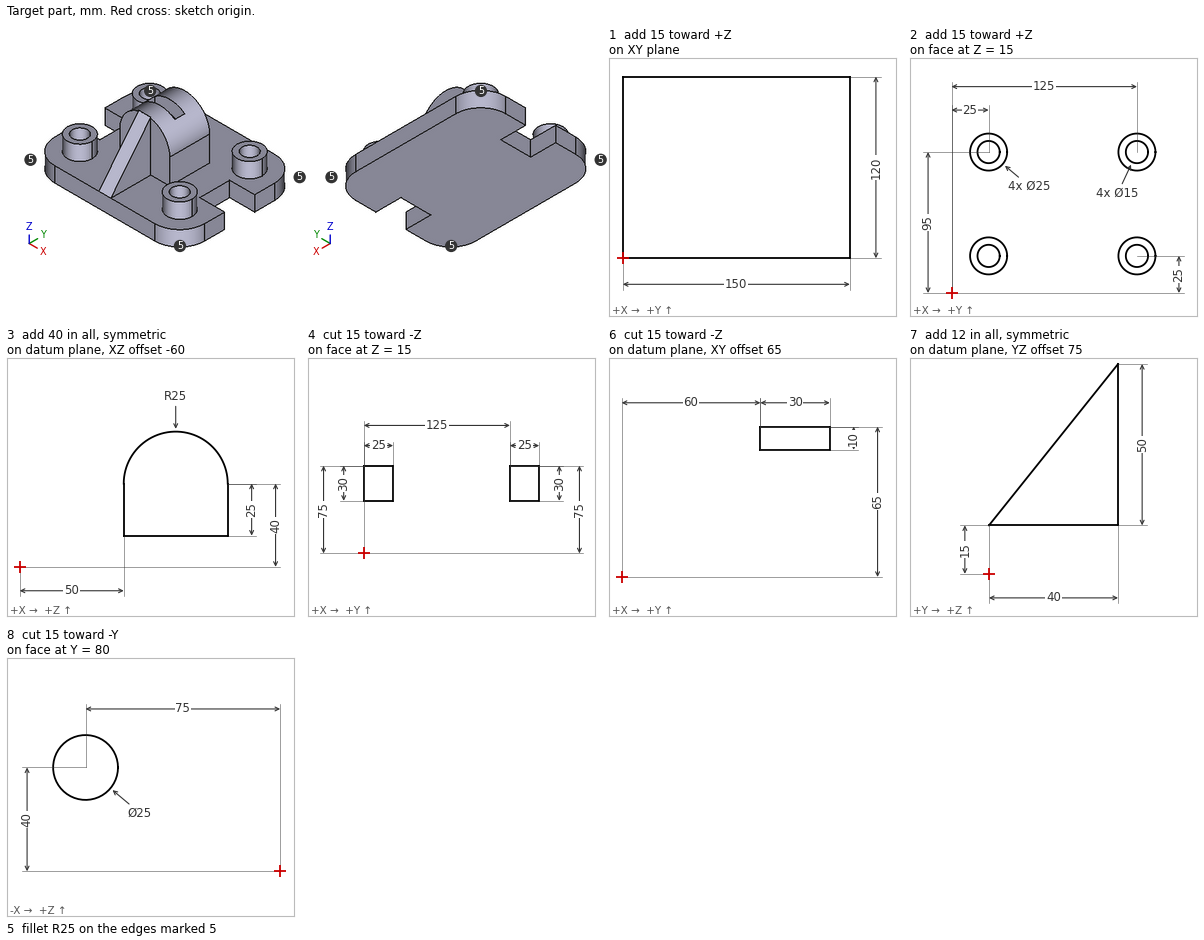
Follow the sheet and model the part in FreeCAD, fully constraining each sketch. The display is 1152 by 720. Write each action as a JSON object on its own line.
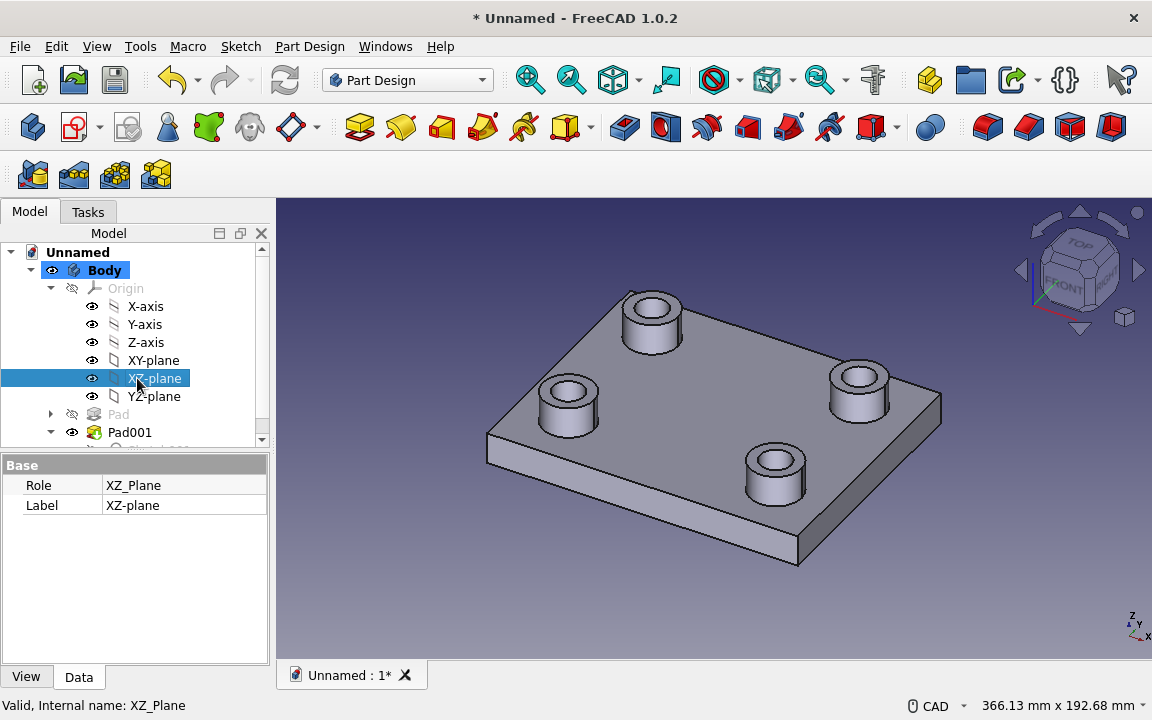
{"action": "left_click", "coordinate": [290, 128]}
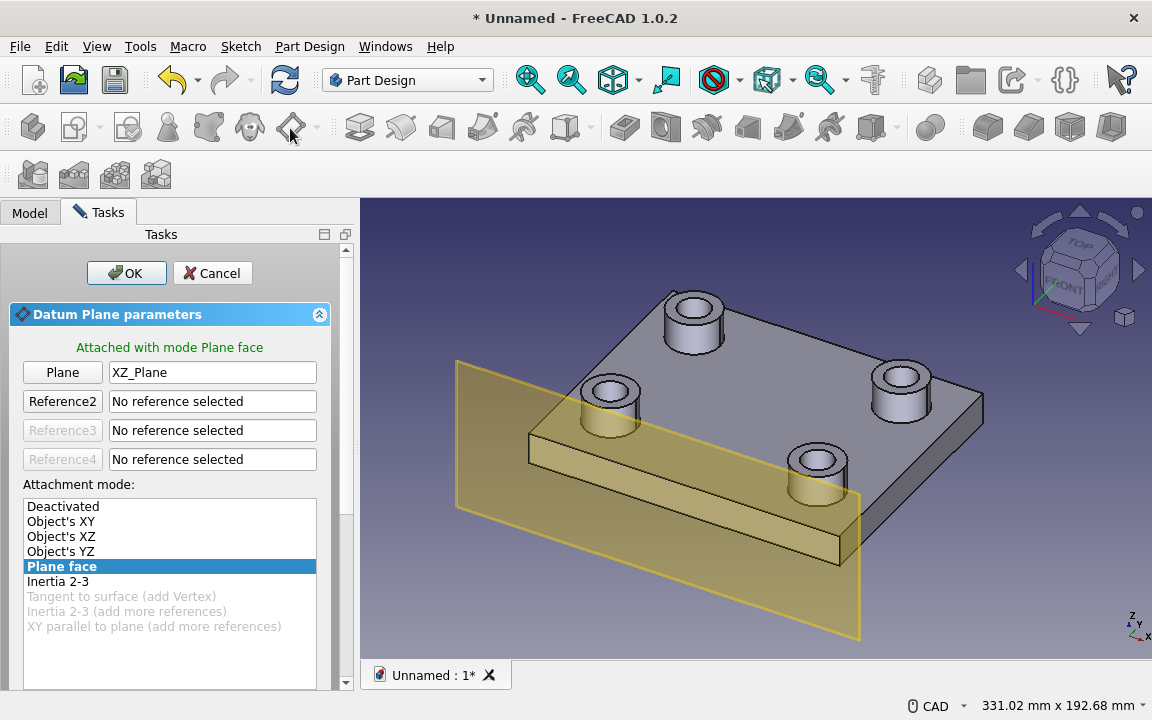
{"action": "scroll", "coordinate": [346, 467], "scroll_direction": "down", "scroll_amount": 4}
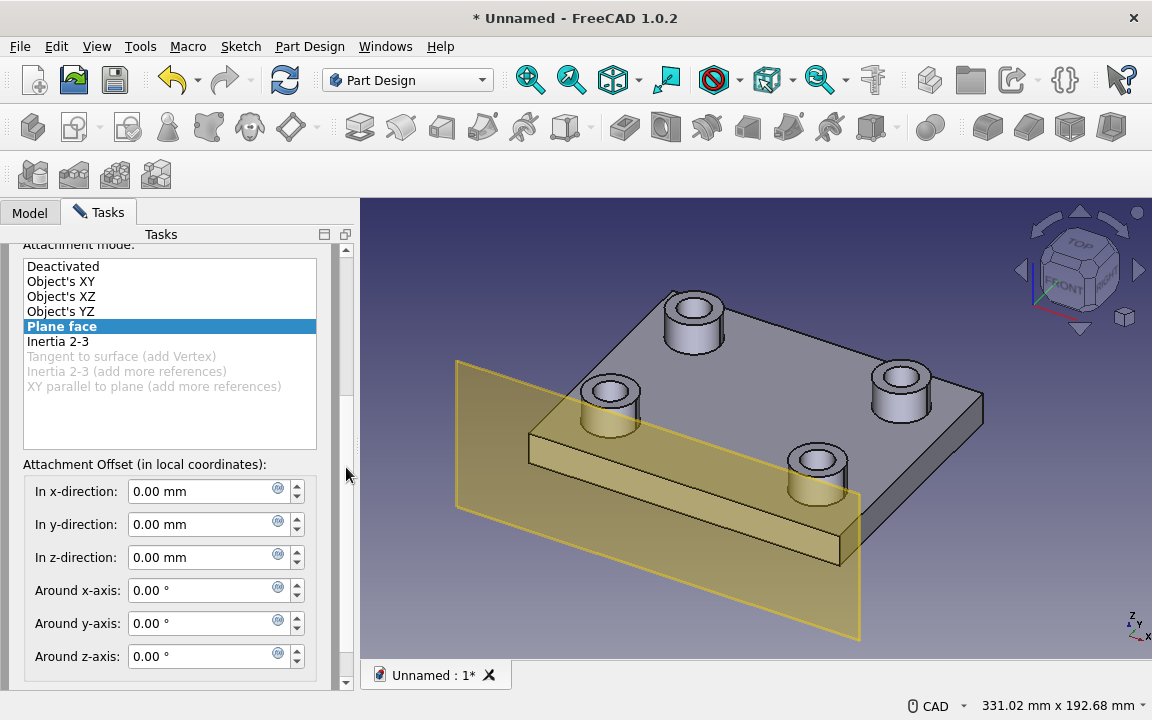
{"action": "triple_click", "coordinate": [210, 558]}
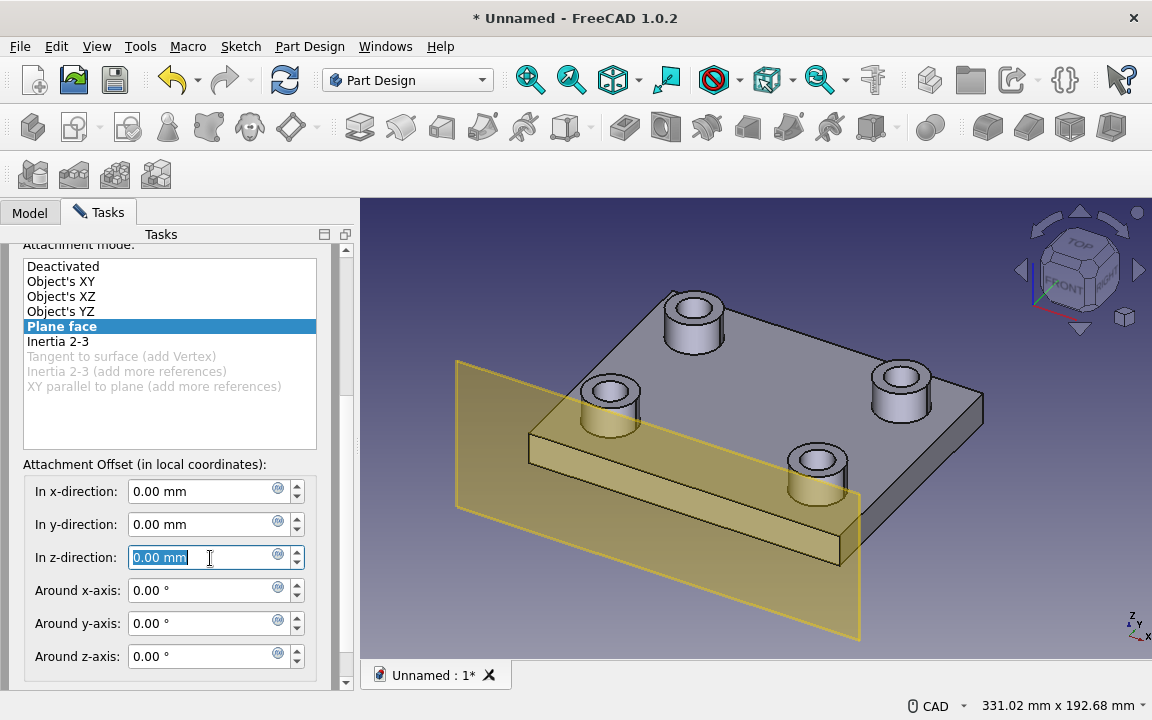
{"action": "type", "text": "-60"}
{"action": "key", "text": "Tab"}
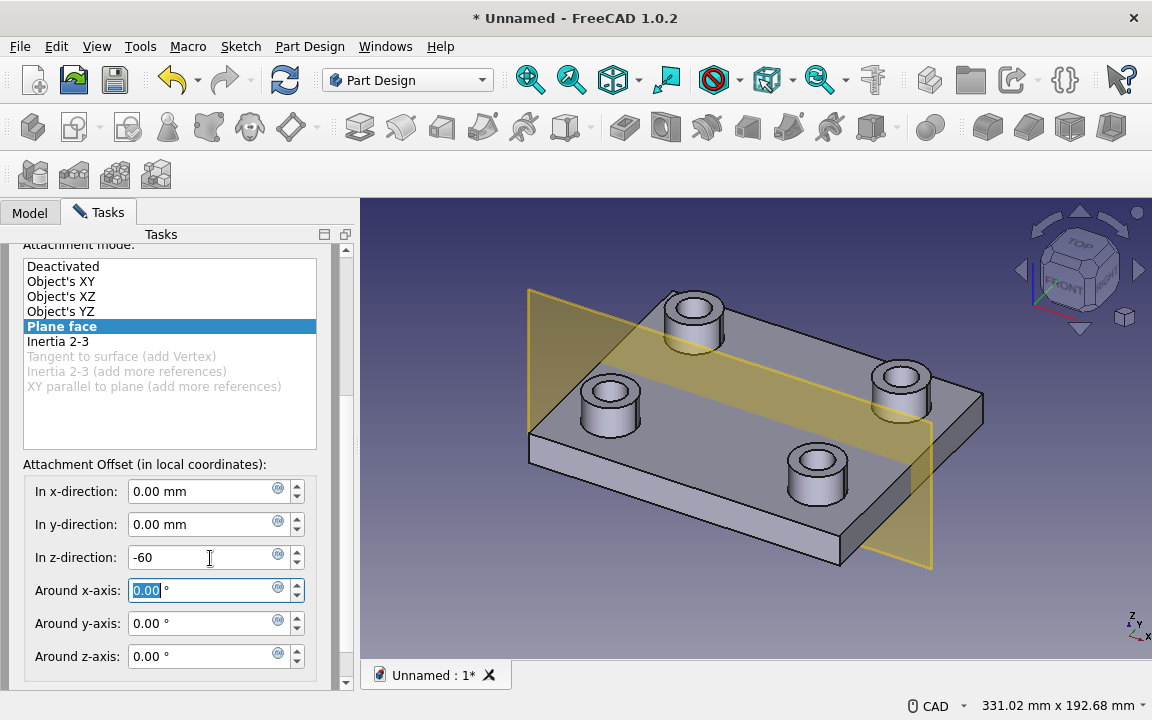
{"action": "scroll", "coordinate": [346, 467], "scroll_direction": "up", "scroll_amount": 5}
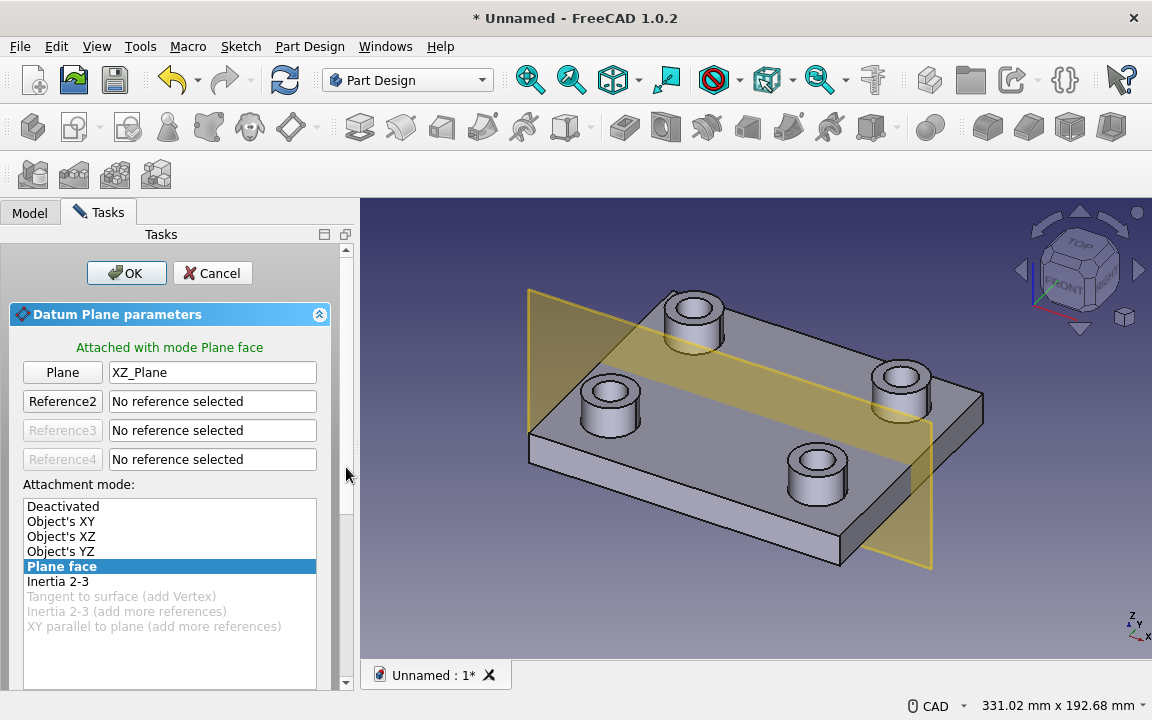
{"action": "left_click", "coordinate": [127, 273]}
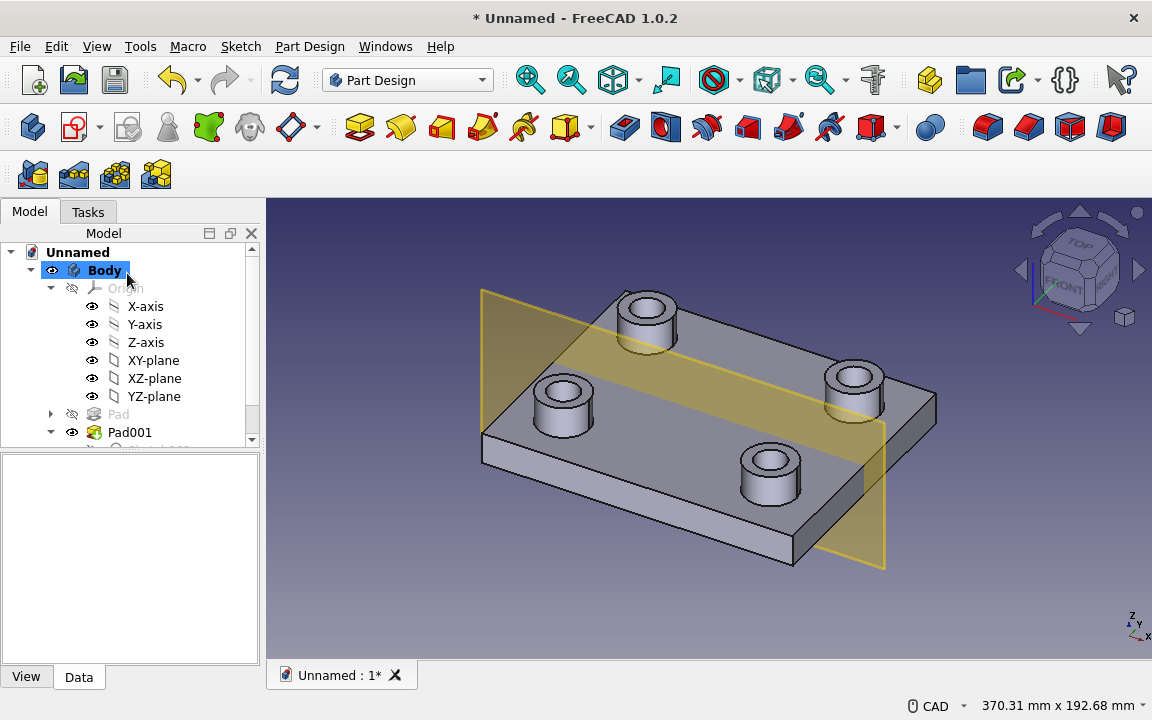
{"action": "scroll", "coordinate": [101, 338], "scroll_direction": "down", "scroll_amount": 3}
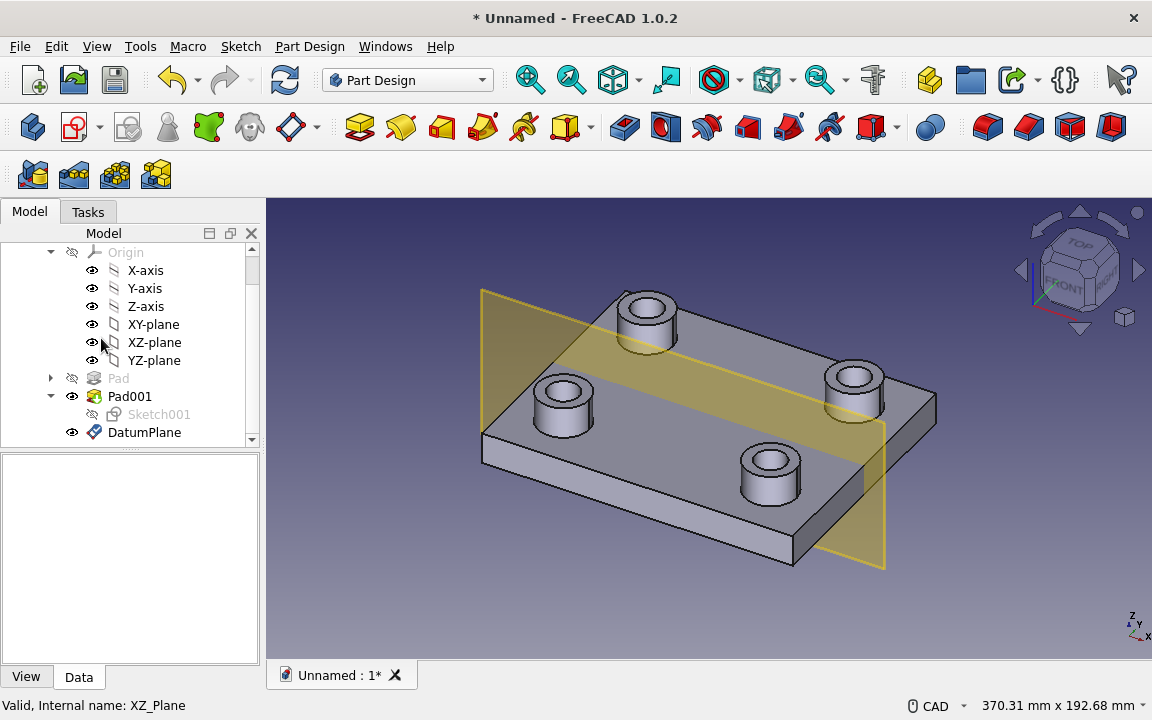
{"action": "left_click", "coordinate": [117, 432]}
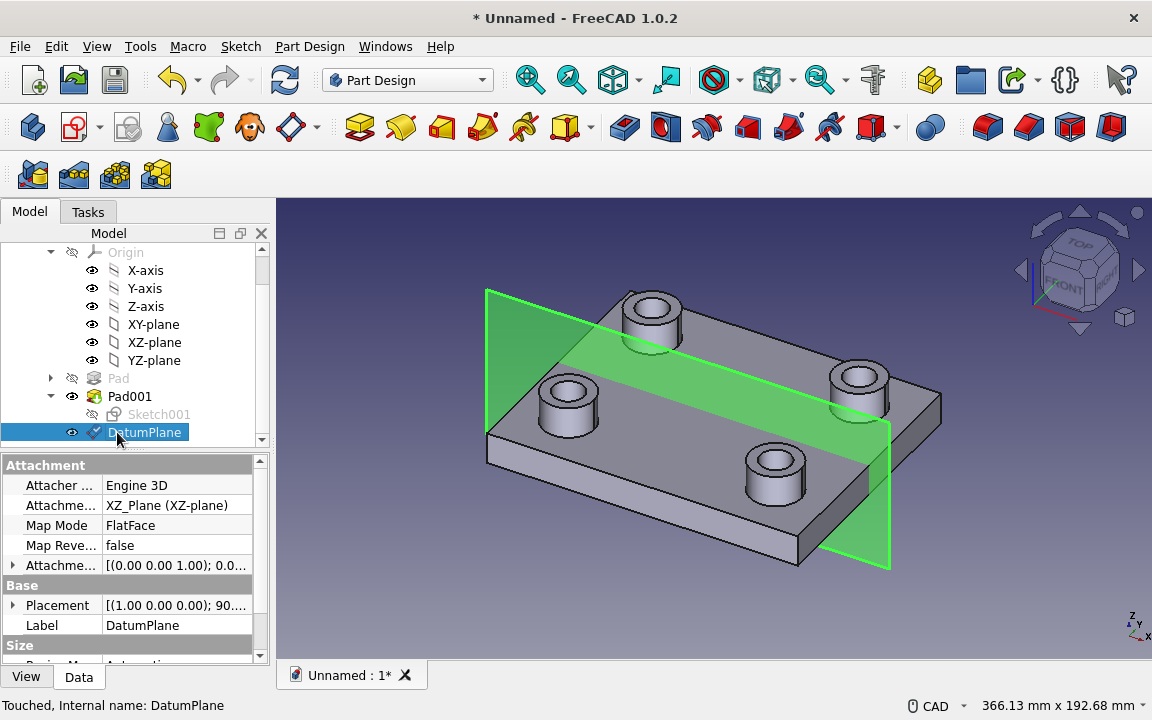
{"action": "left_click", "coordinate": [74, 128]}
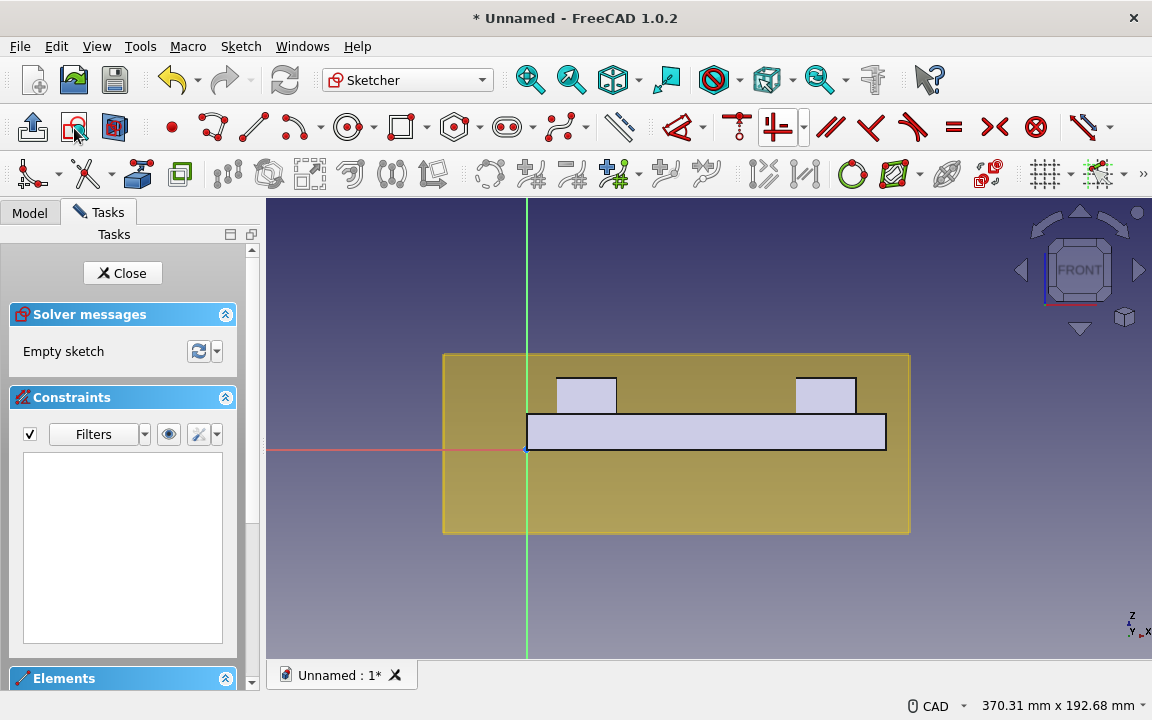
{"action": "left_click", "coordinate": [115, 128]}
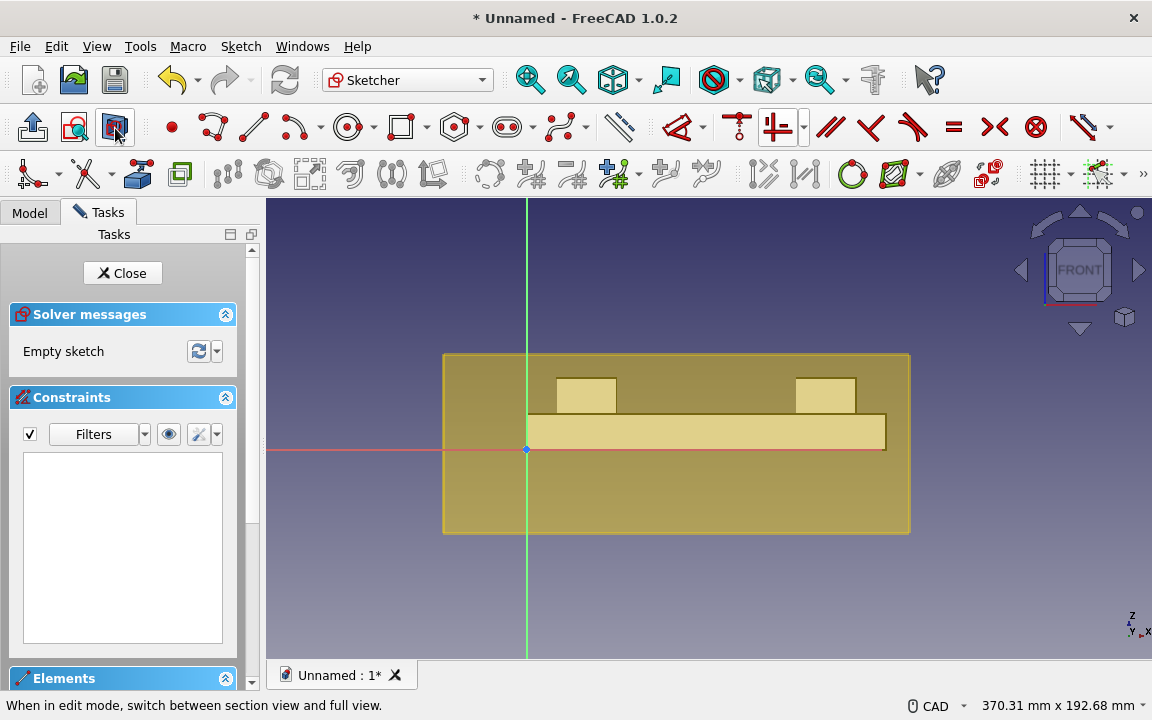
{"action": "scroll", "coordinate": [654, 304], "scroll_direction": "up", "scroll_amount": 3}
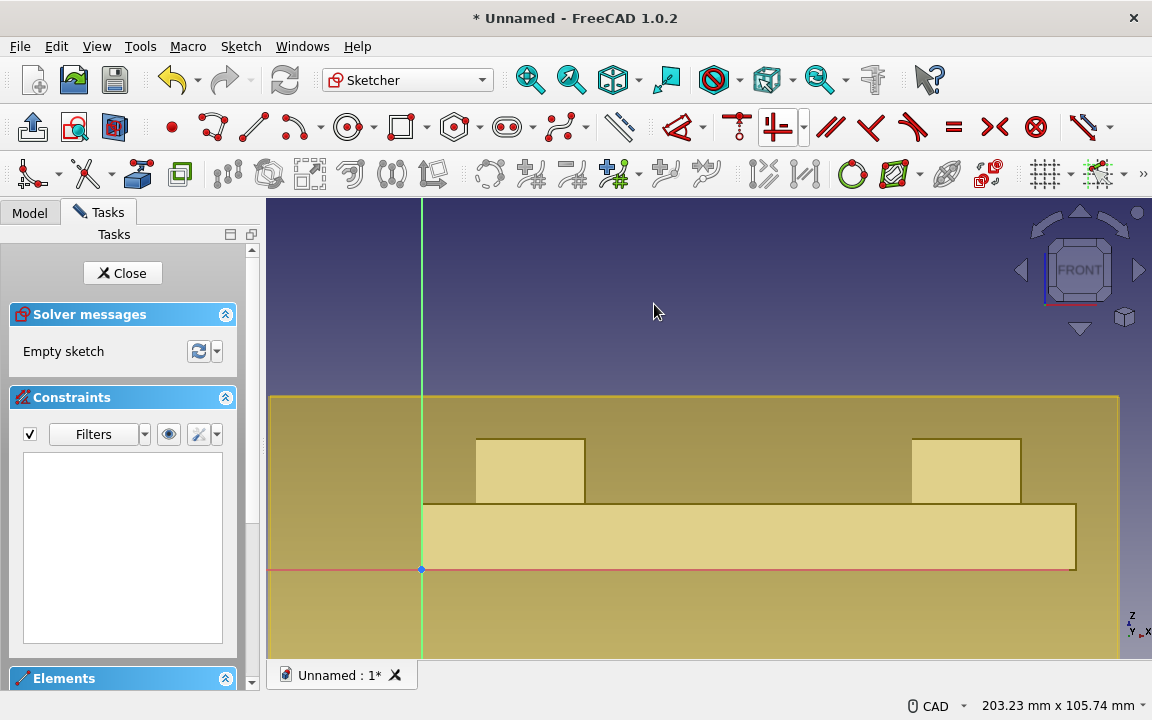
{"action": "left_click", "coordinate": [213, 128]}